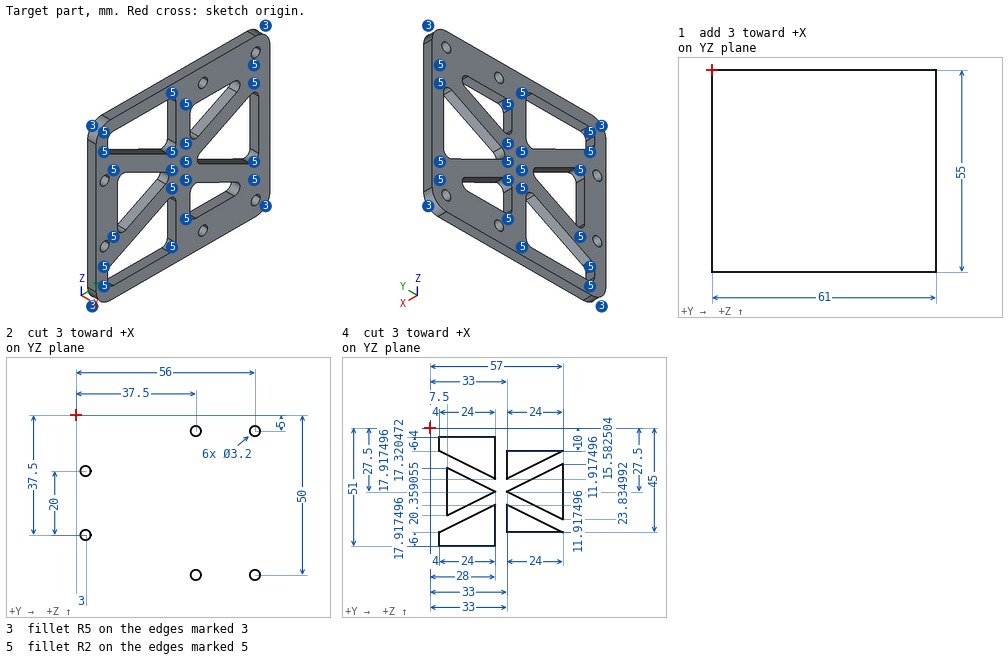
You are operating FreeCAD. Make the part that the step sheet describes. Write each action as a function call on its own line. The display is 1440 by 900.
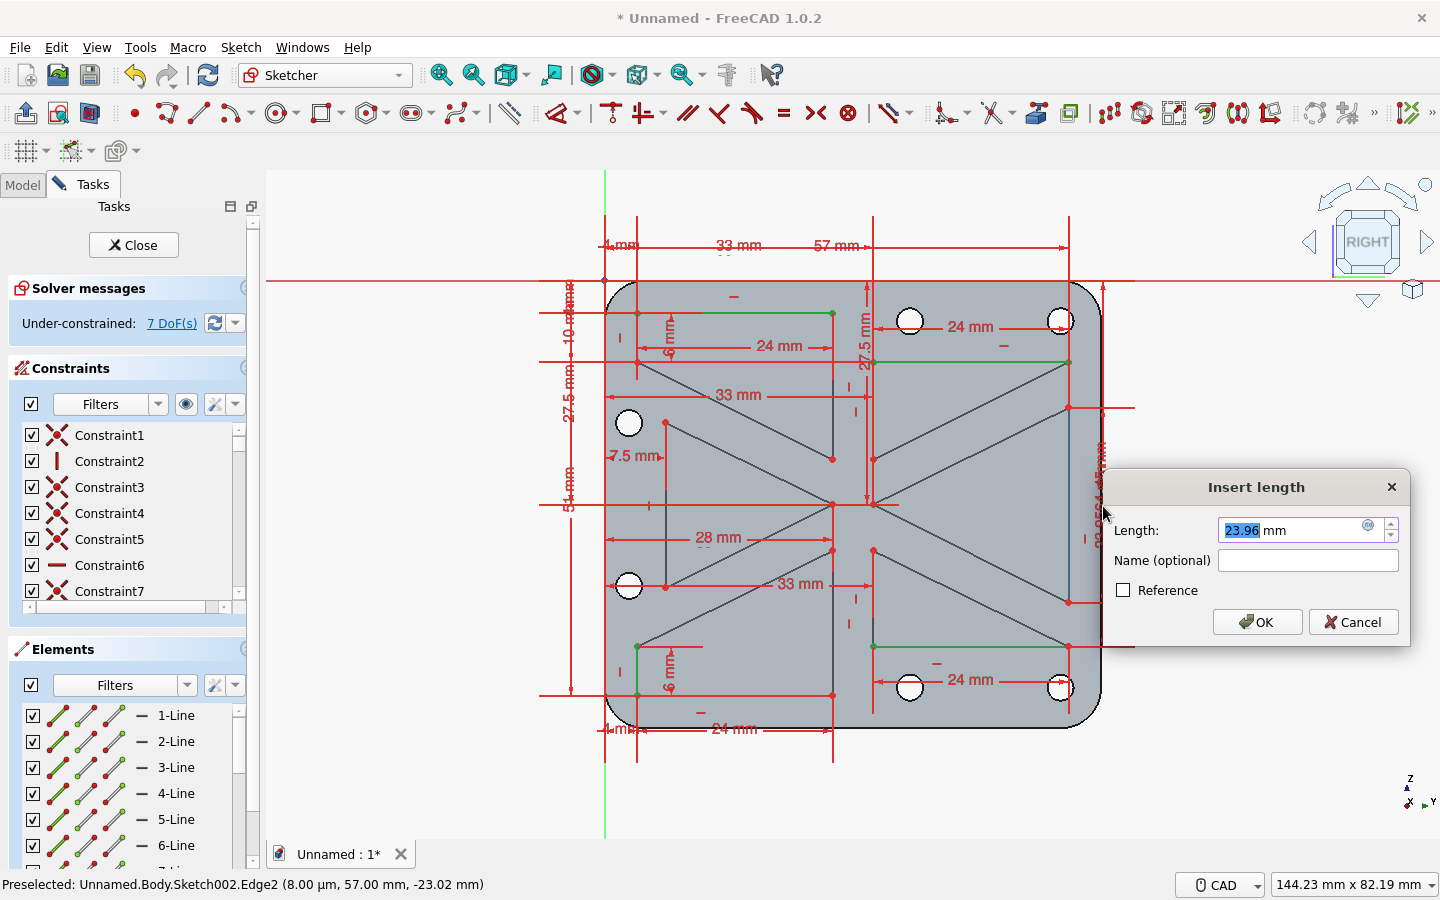
text(23.834992)
key(Return)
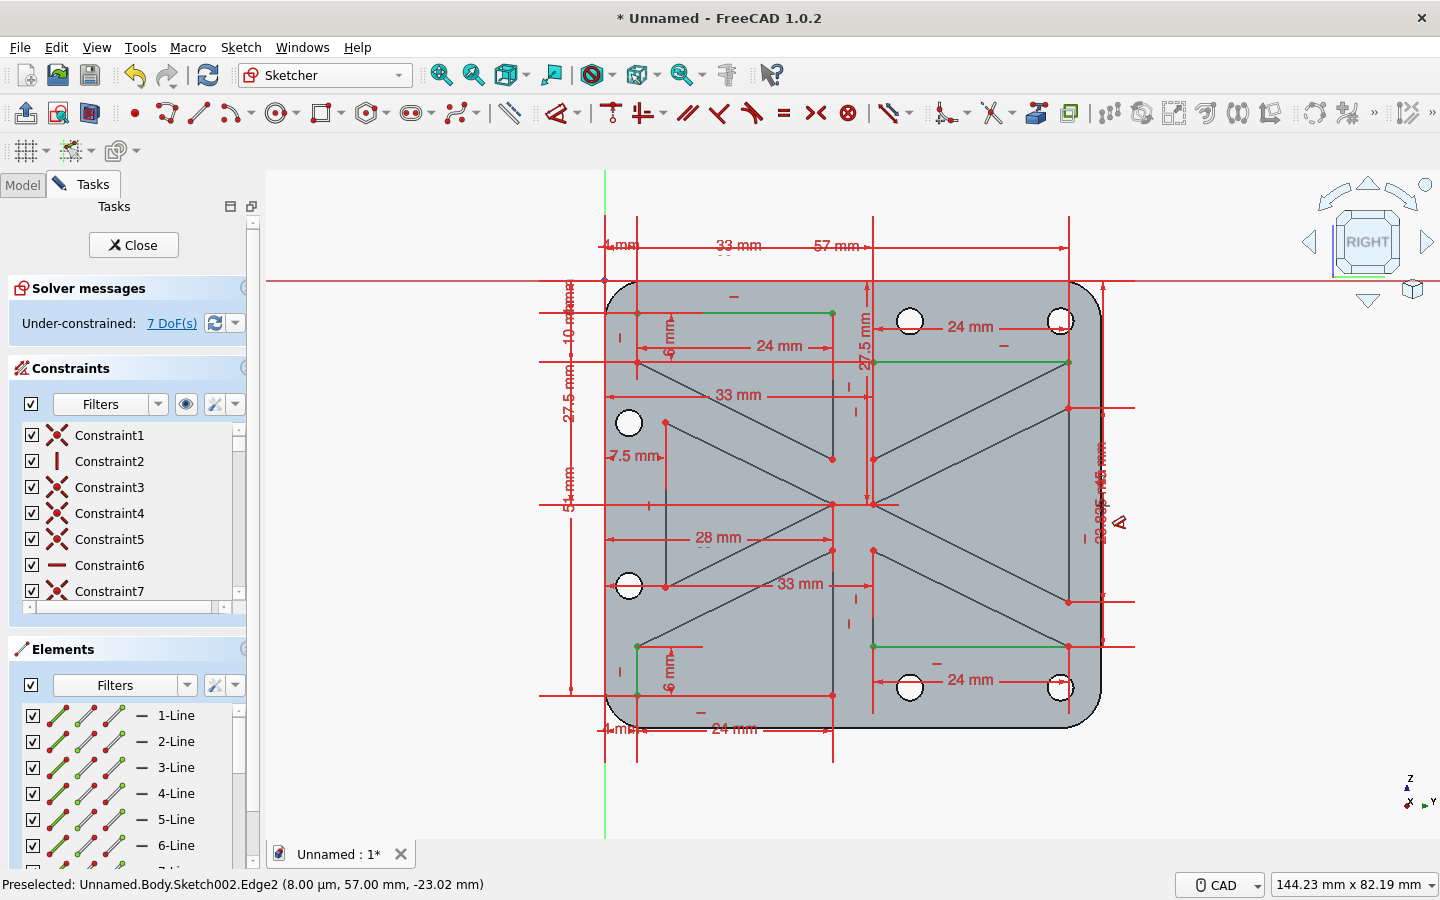
click(873, 618)
click(907, 599)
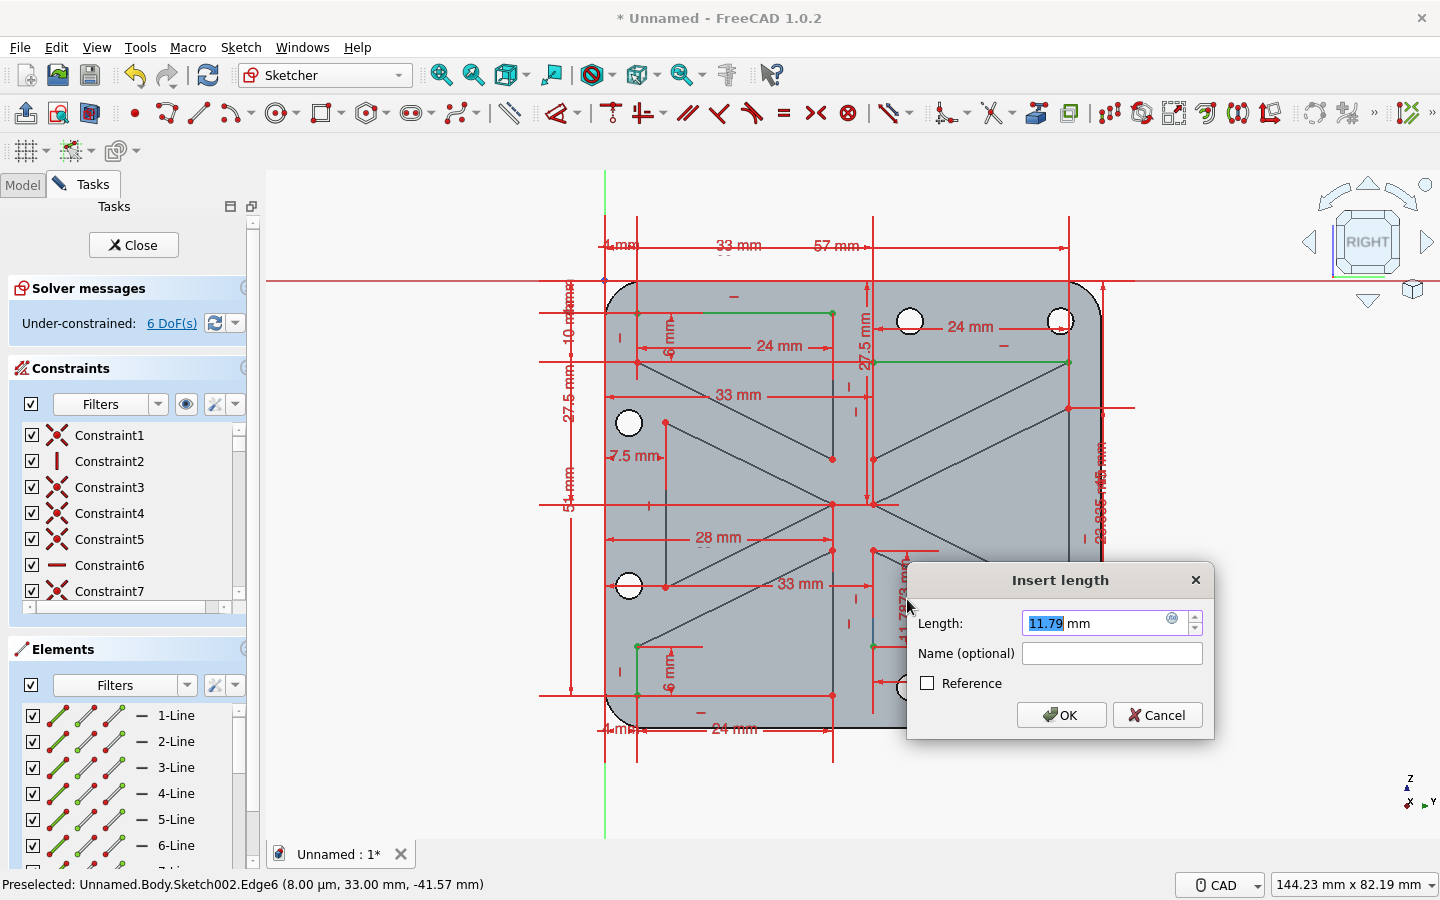
text(11.917496)
key(Return)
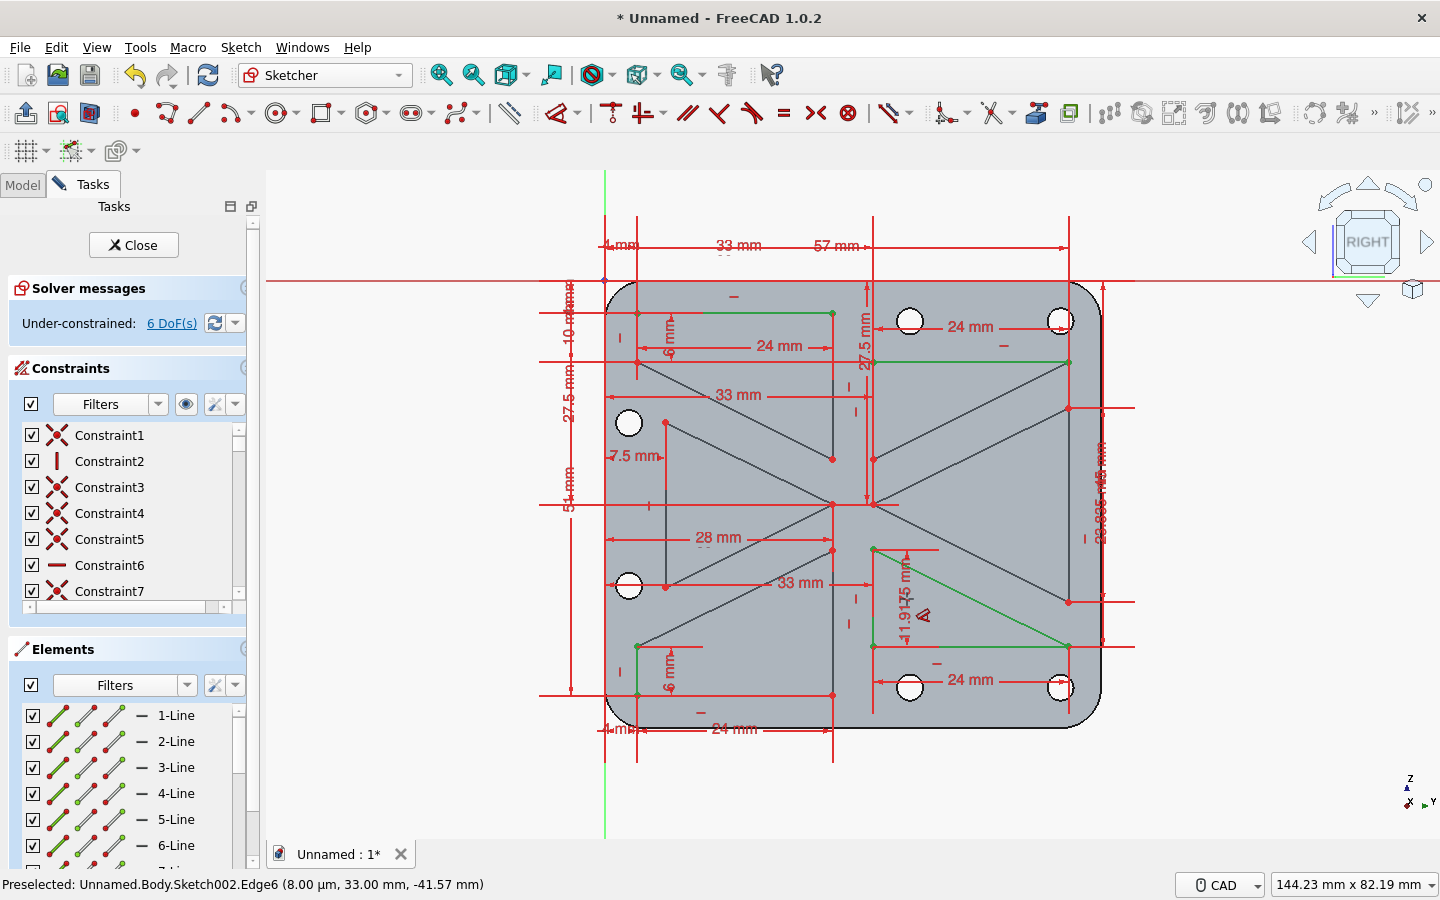
click(873, 431)
click(907, 411)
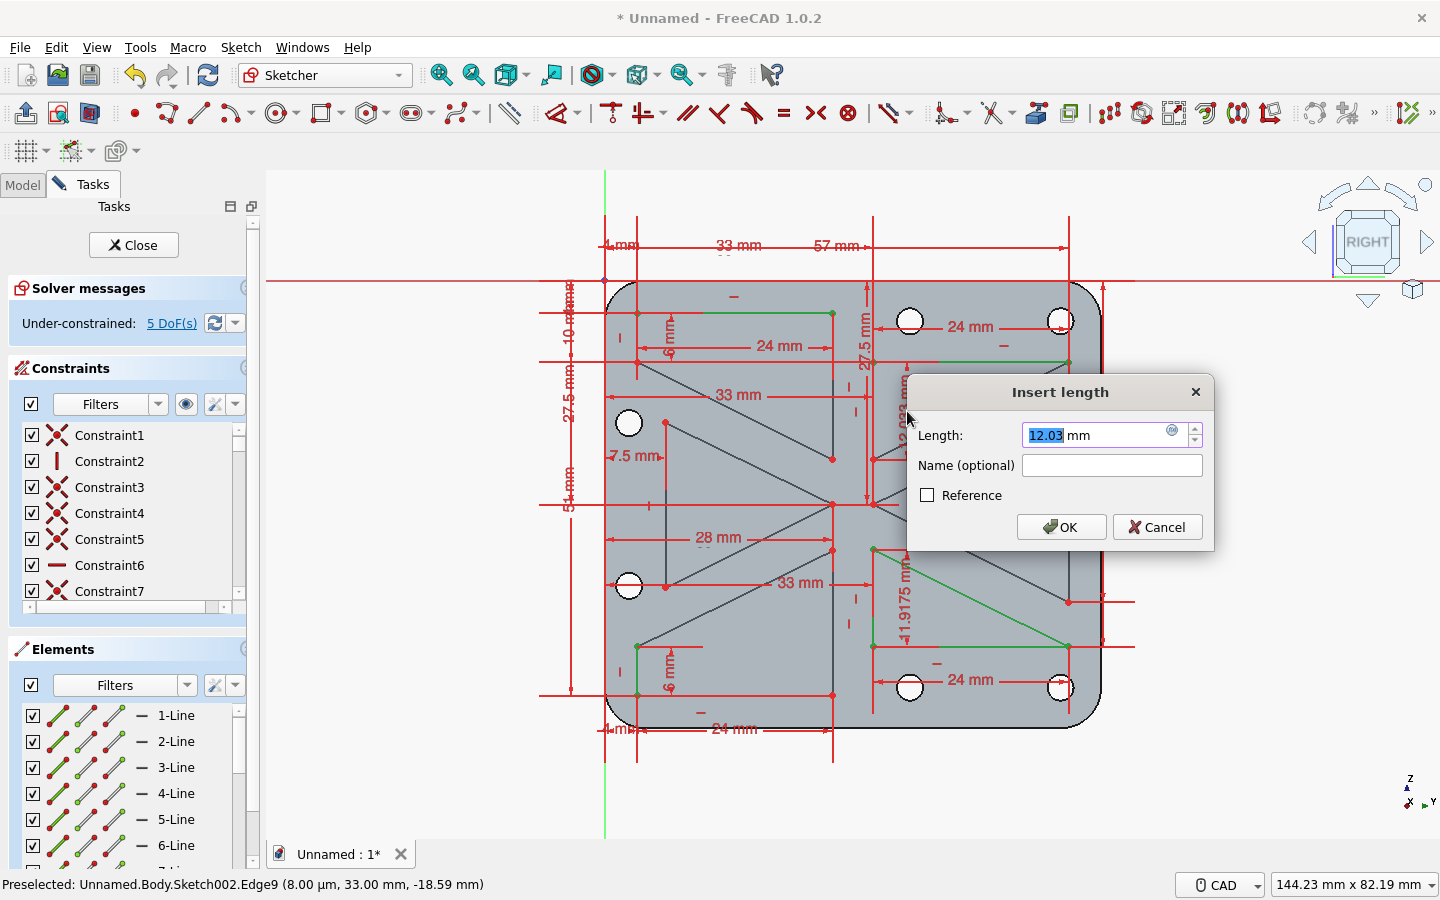
text(11.917496)
key(Return)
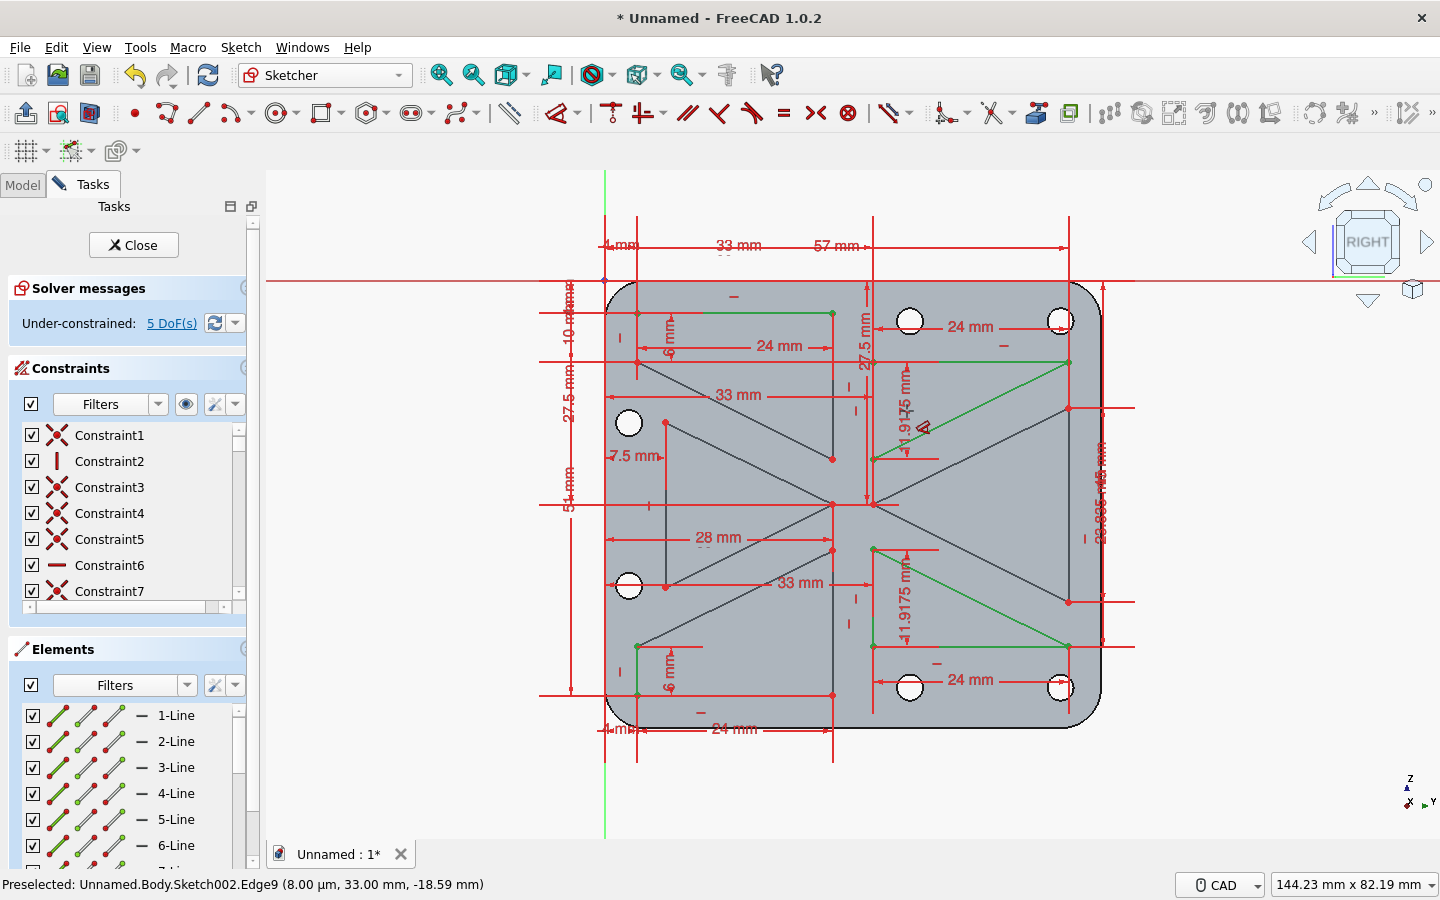
click(833, 357)
click(799, 420)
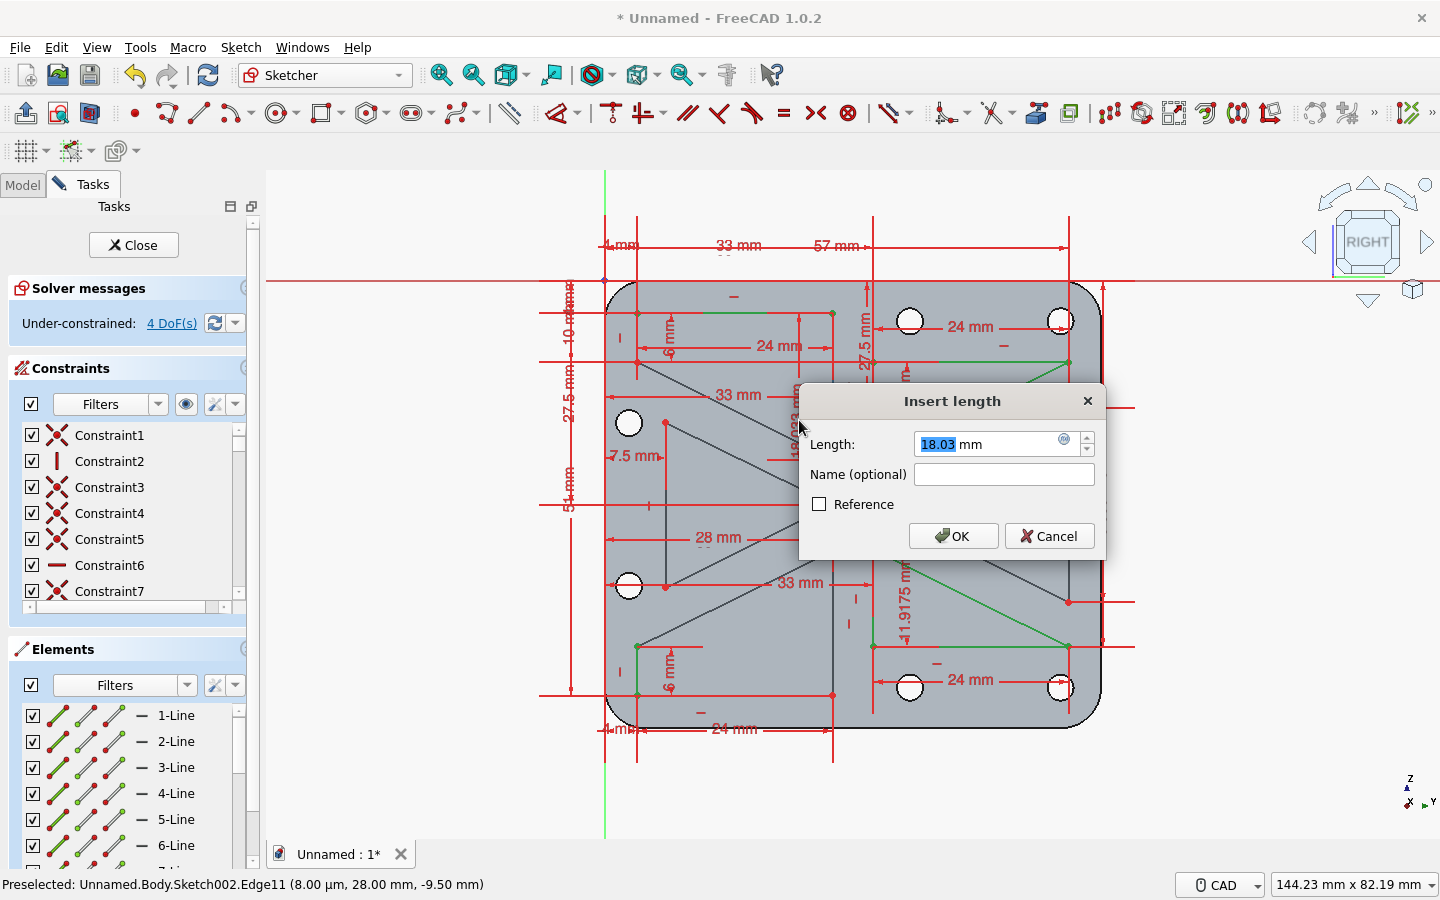
text(17.917496)
key(Return)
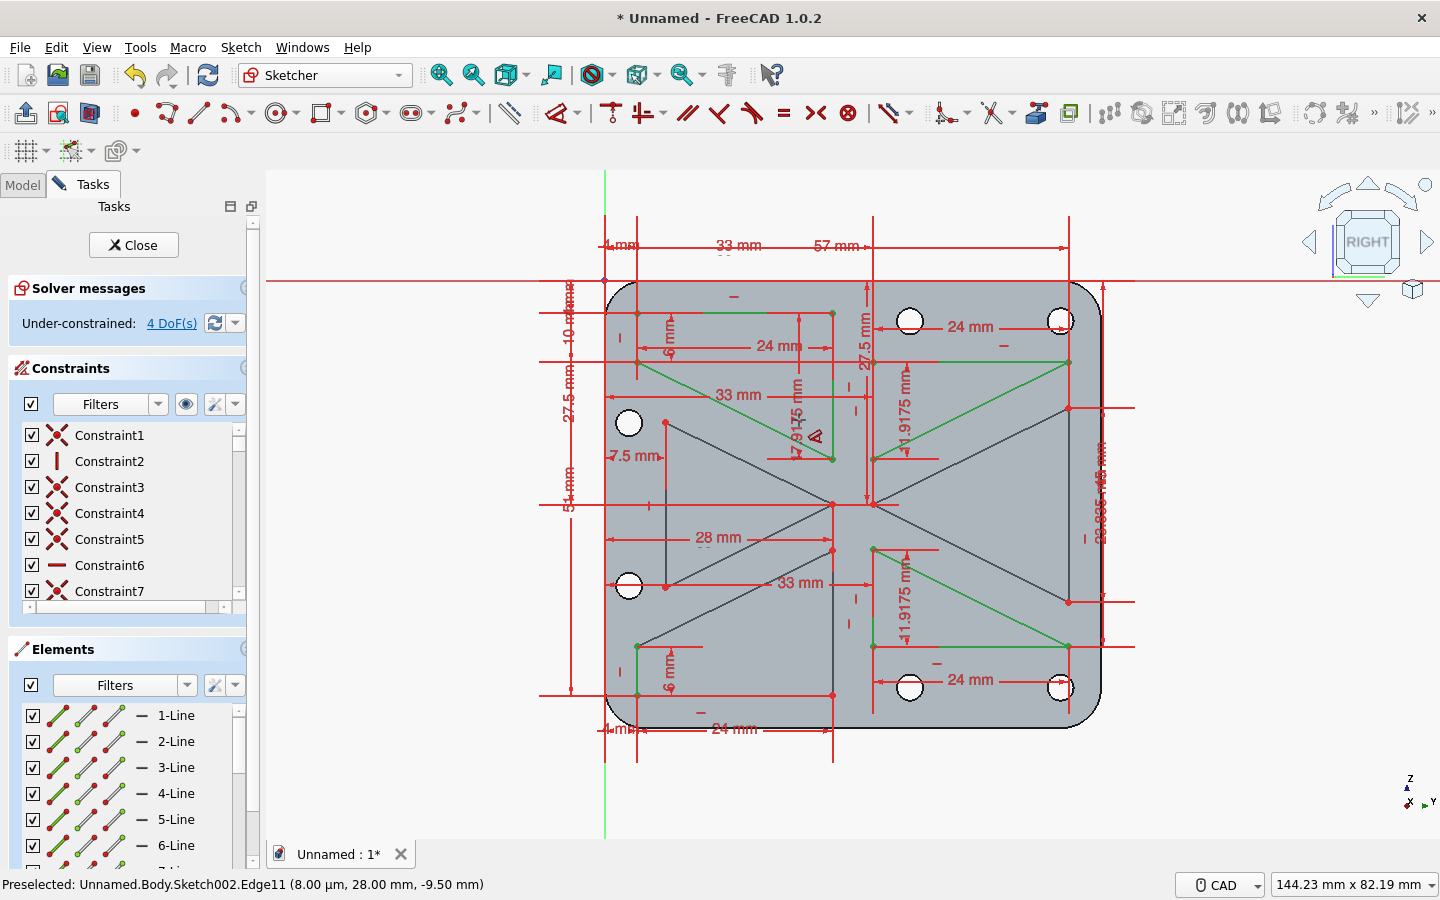
click(666, 538)
click(632, 543)